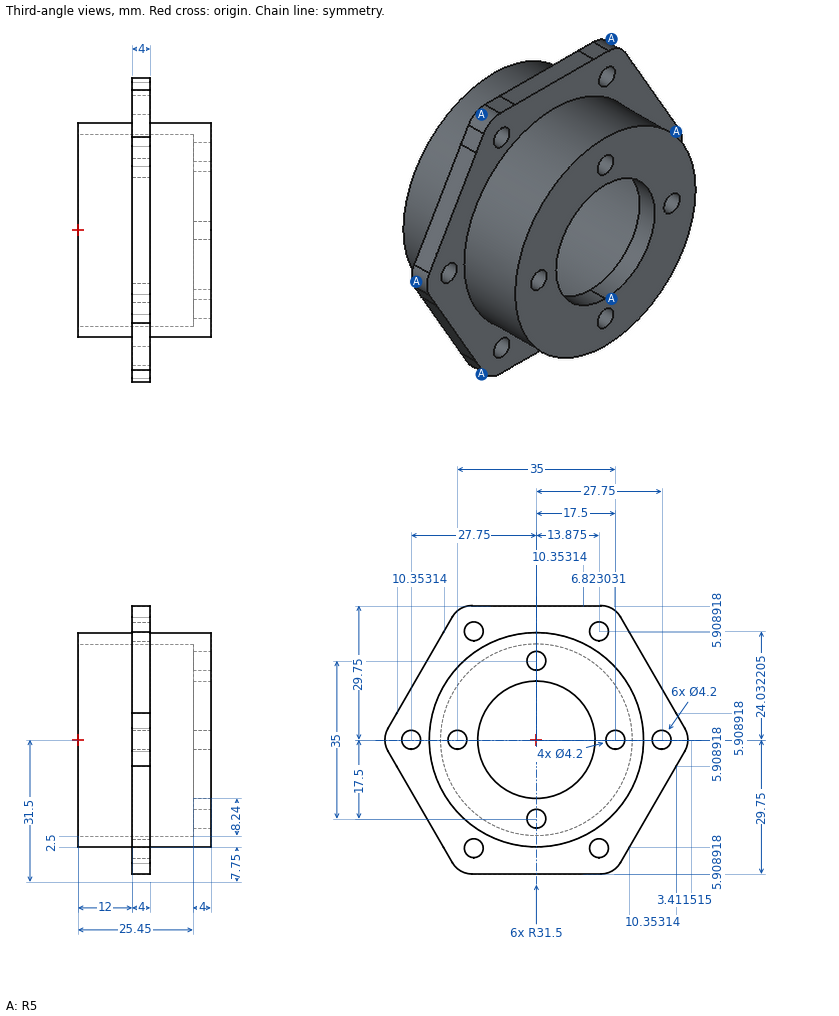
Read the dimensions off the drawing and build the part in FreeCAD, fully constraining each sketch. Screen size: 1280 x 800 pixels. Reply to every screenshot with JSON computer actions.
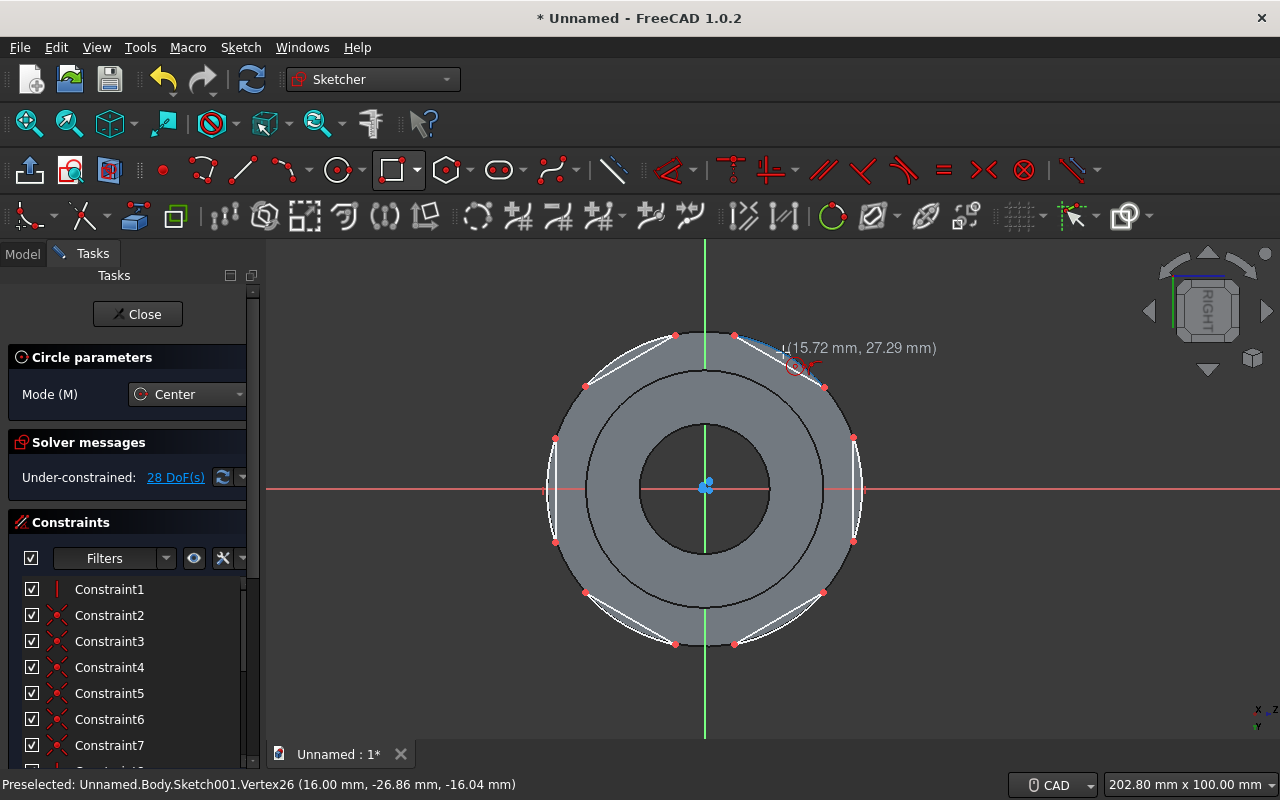
{"action": "scroll", "coordinate": [705, 628], "scroll_direction": "up", "scroll_amount": 4}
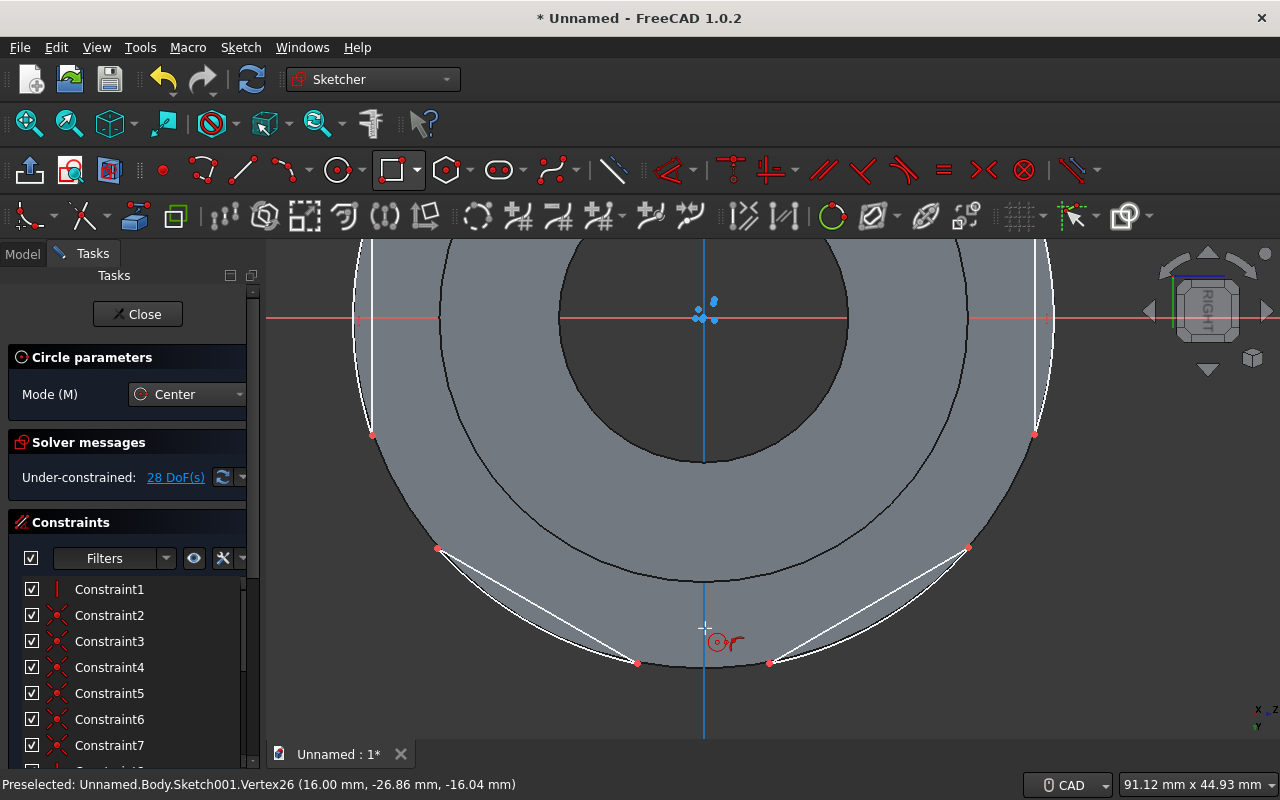
{"action": "left_click", "coordinate": [704, 627]}
{"action": "left_click", "coordinate": [720, 610]}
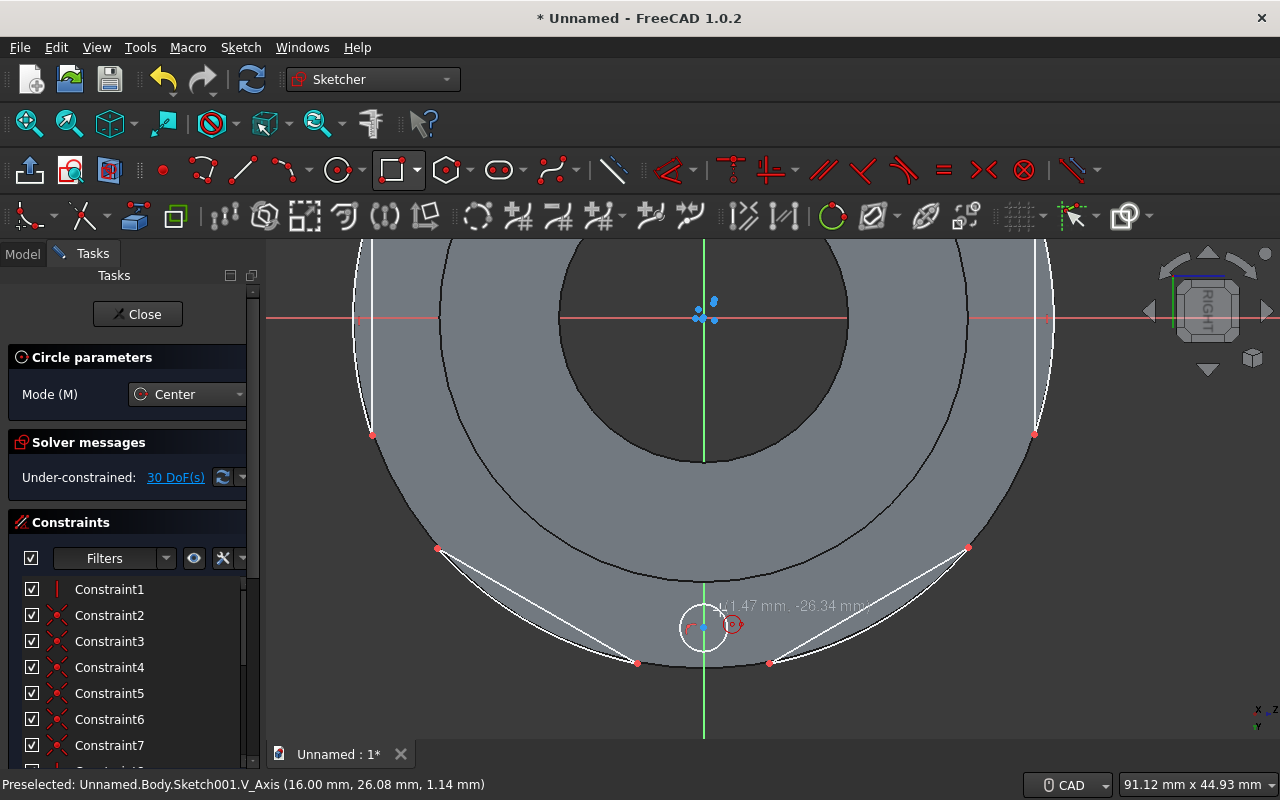
{"action": "left_click", "coordinate": [971, 472]}
{"action": "left_click", "coordinate": [988, 456]}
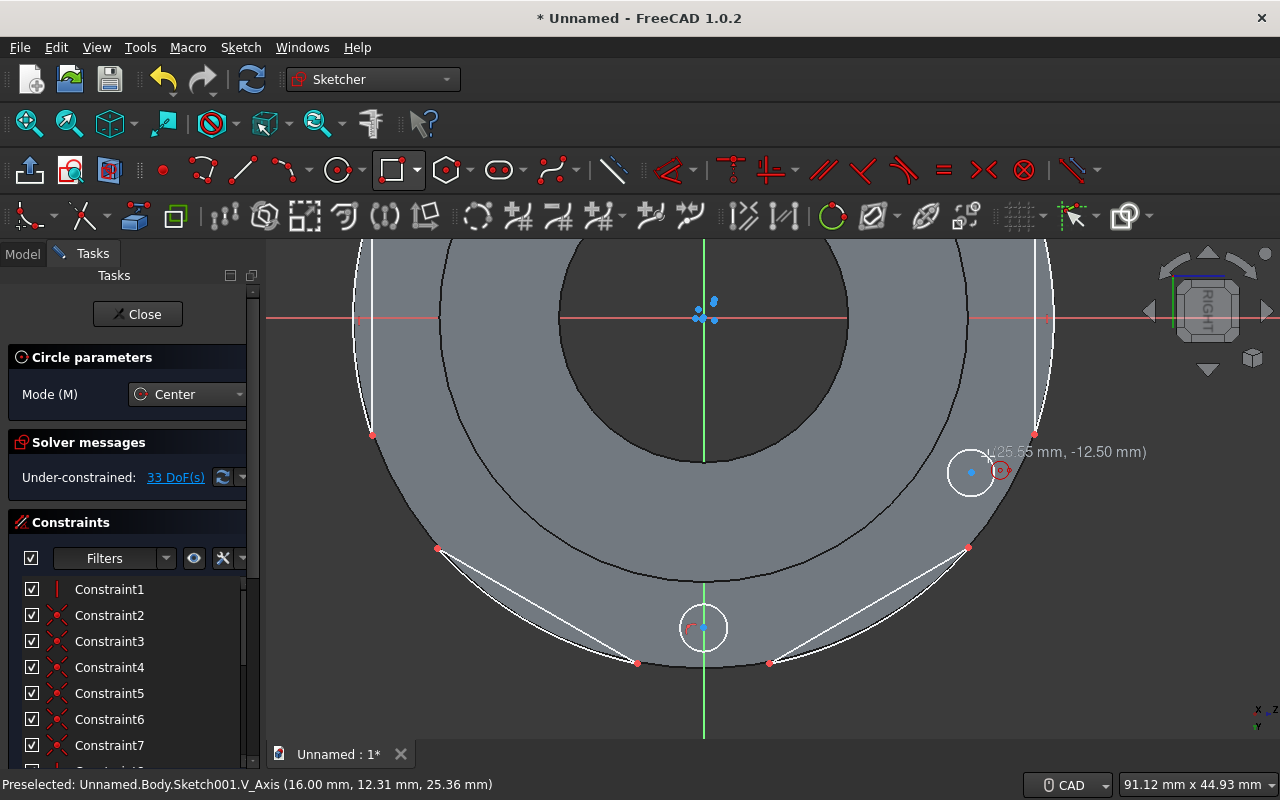
{"action": "scroll", "coordinate": [705, 629], "scroll_direction": "down", "scroll_amount": 4}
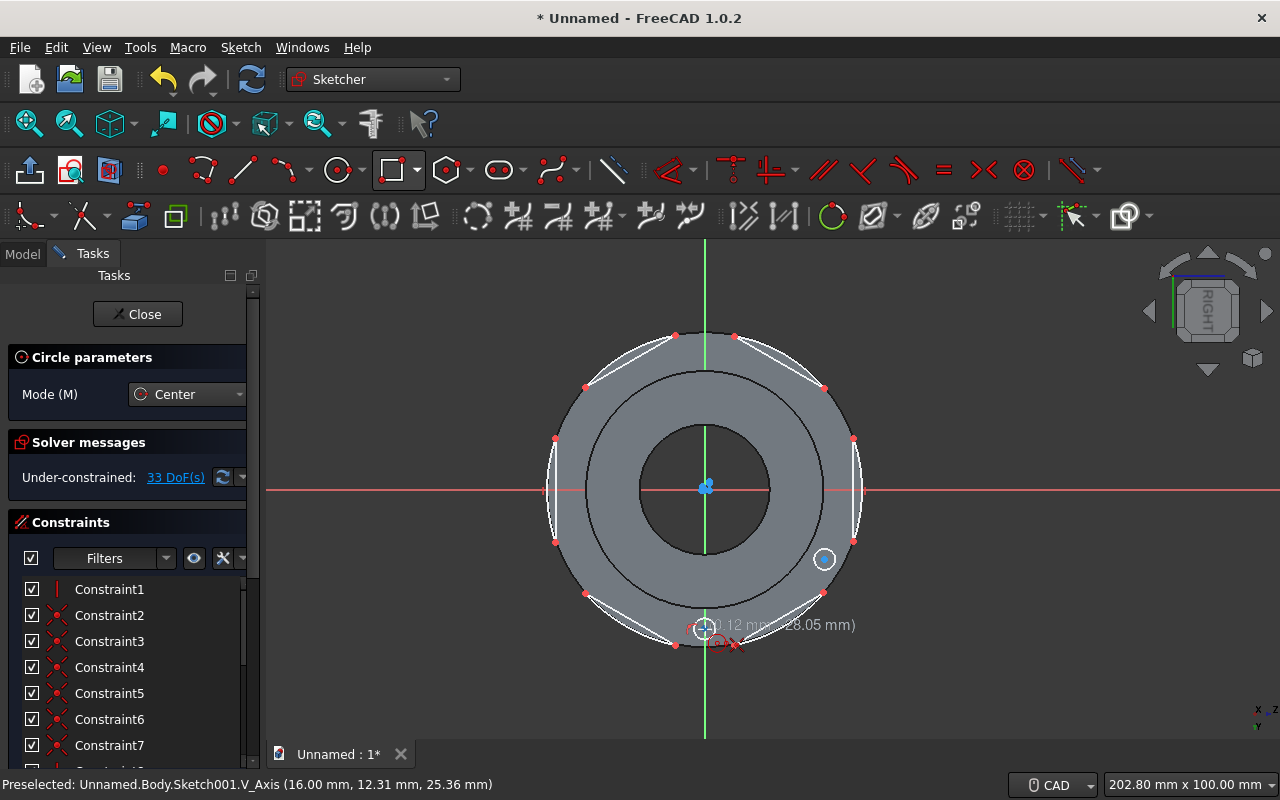
{"action": "scroll", "coordinate": [825, 420], "scroll_direction": "up", "scroll_amount": 4}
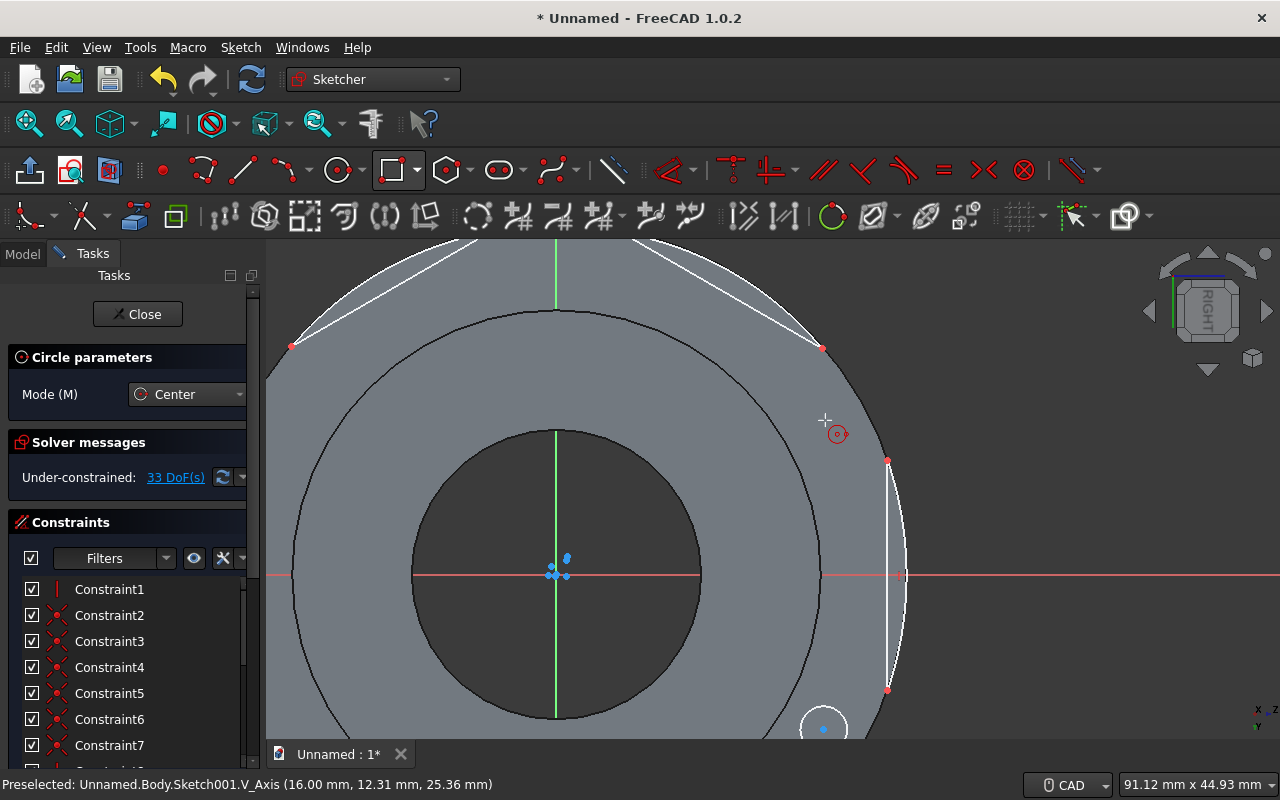
{"action": "left_click", "coordinate": [824, 420]}
{"action": "left_click", "coordinate": [840, 404]}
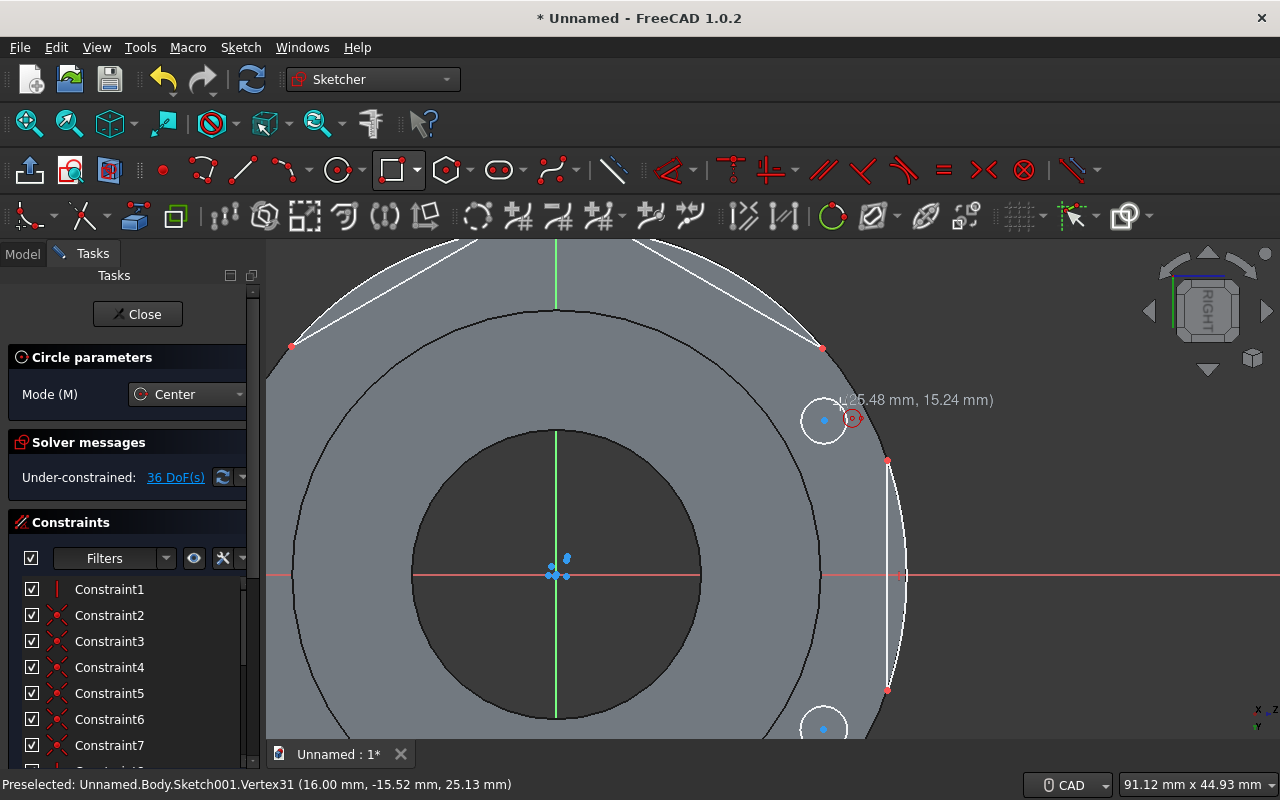
{"action": "scroll", "coordinate": [825, 419], "scroll_direction": "down", "scroll_amount": 4}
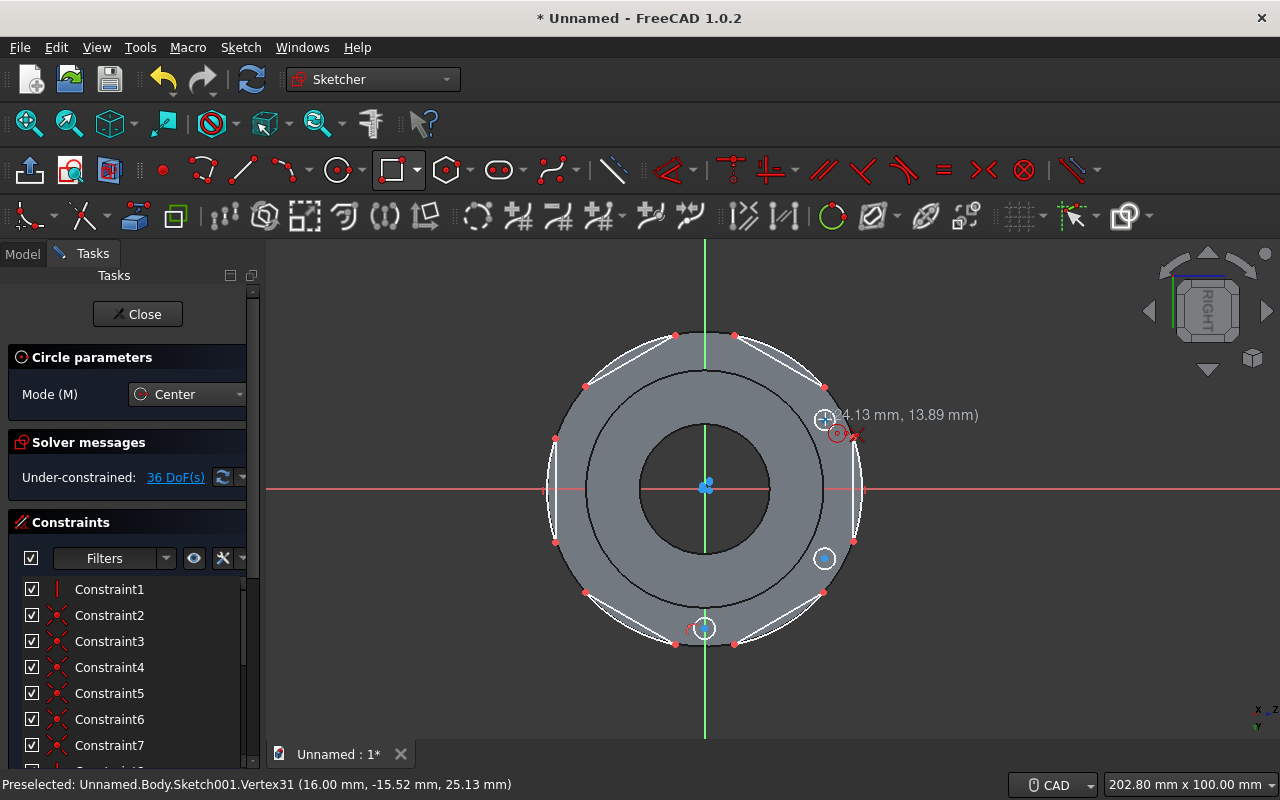
{"action": "scroll", "coordinate": [705, 350], "scroll_direction": "up", "scroll_amount": 4}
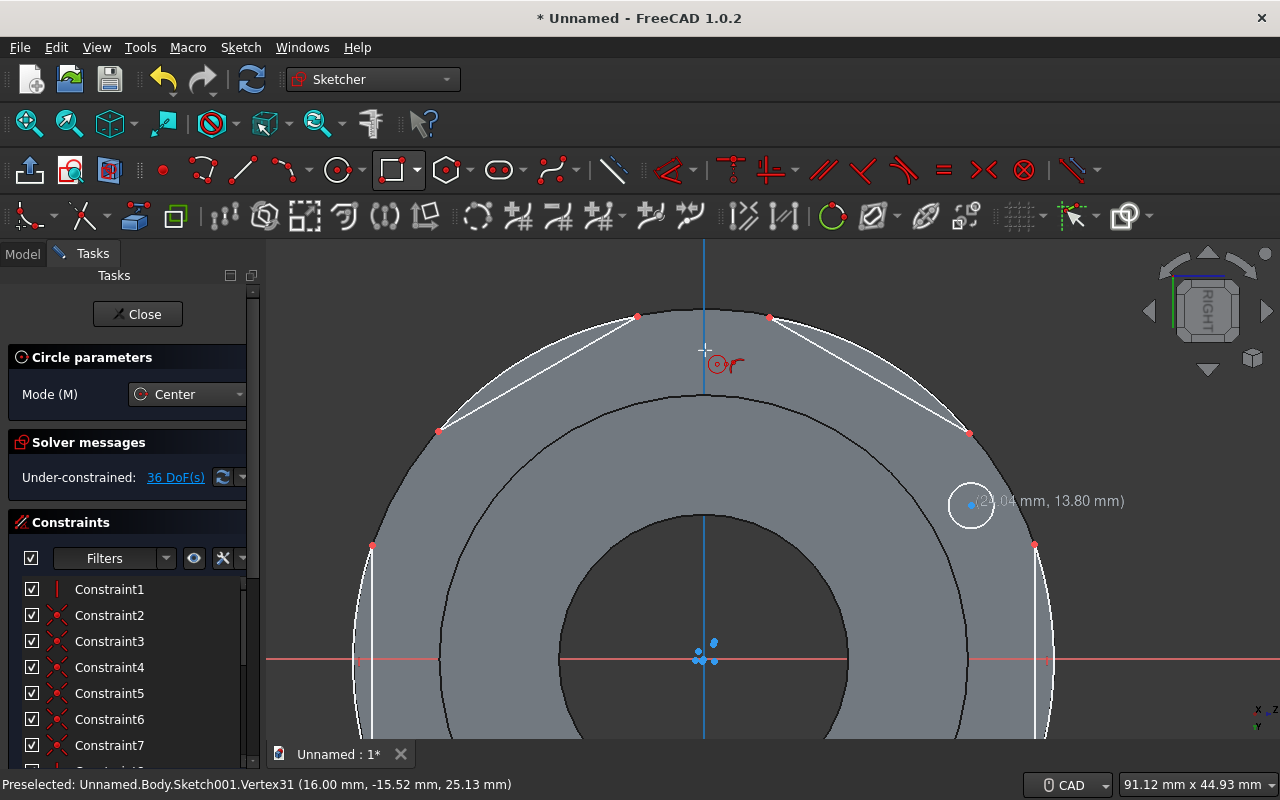
{"action": "left_click", "coordinate": [704, 351]}
{"action": "left_click", "coordinate": [720, 334]}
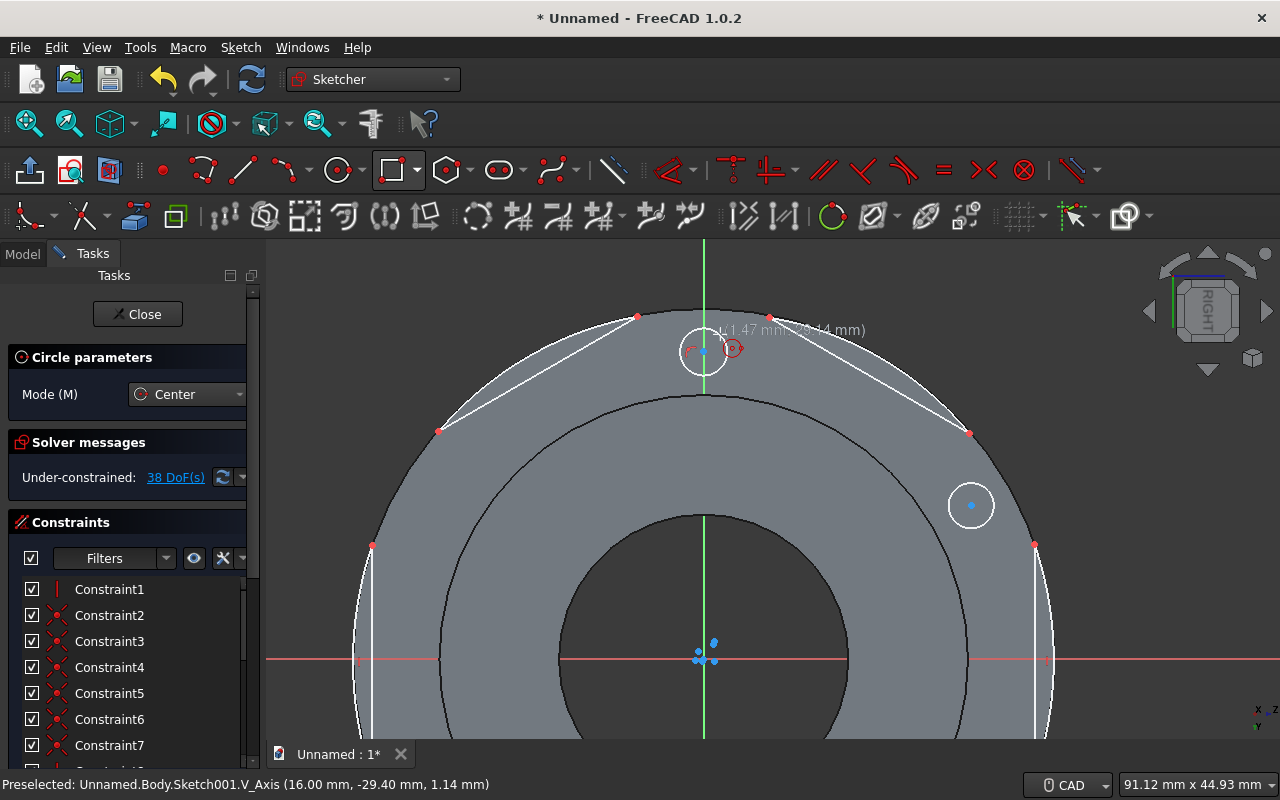
{"action": "left_click", "coordinate": [436, 505]}
{"action": "left_click", "coordinate": [453, 488]}